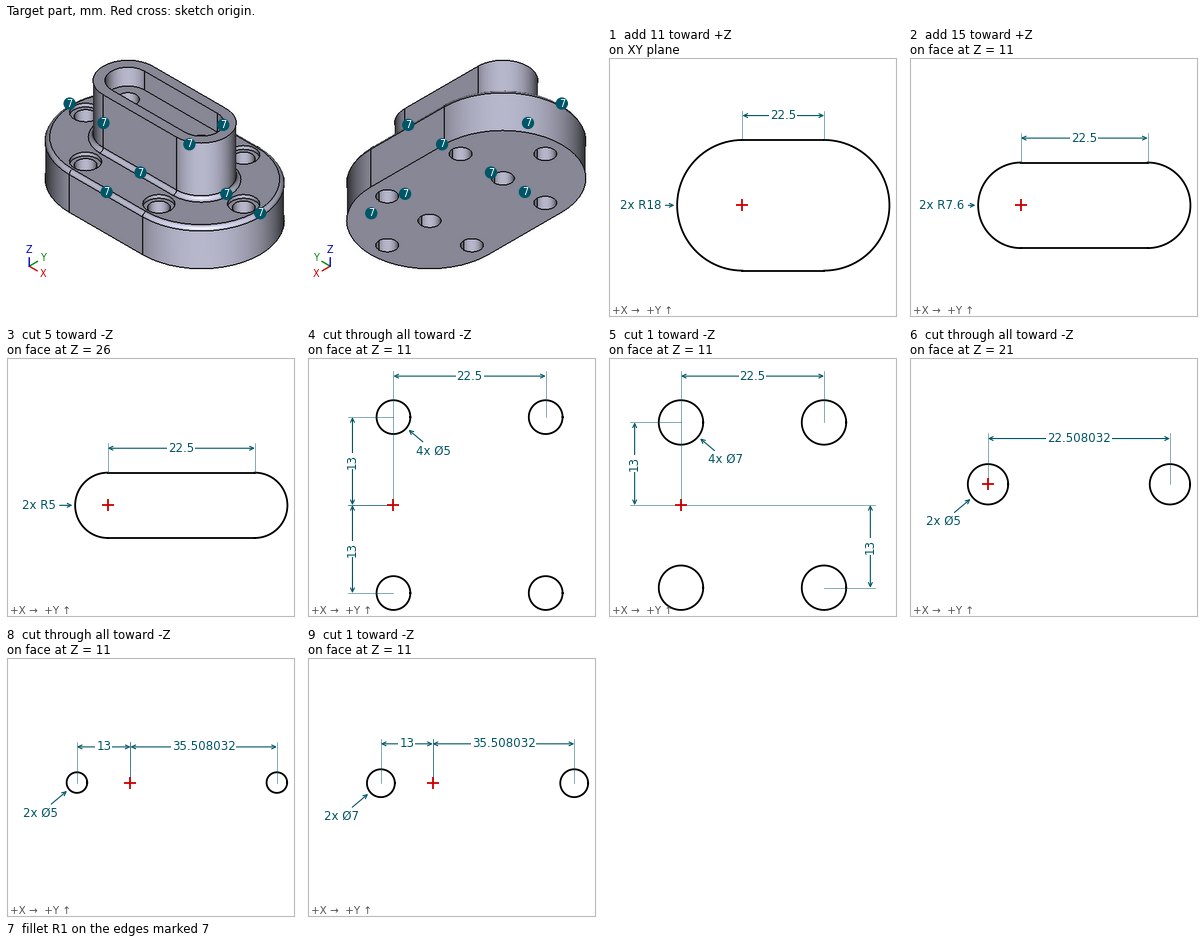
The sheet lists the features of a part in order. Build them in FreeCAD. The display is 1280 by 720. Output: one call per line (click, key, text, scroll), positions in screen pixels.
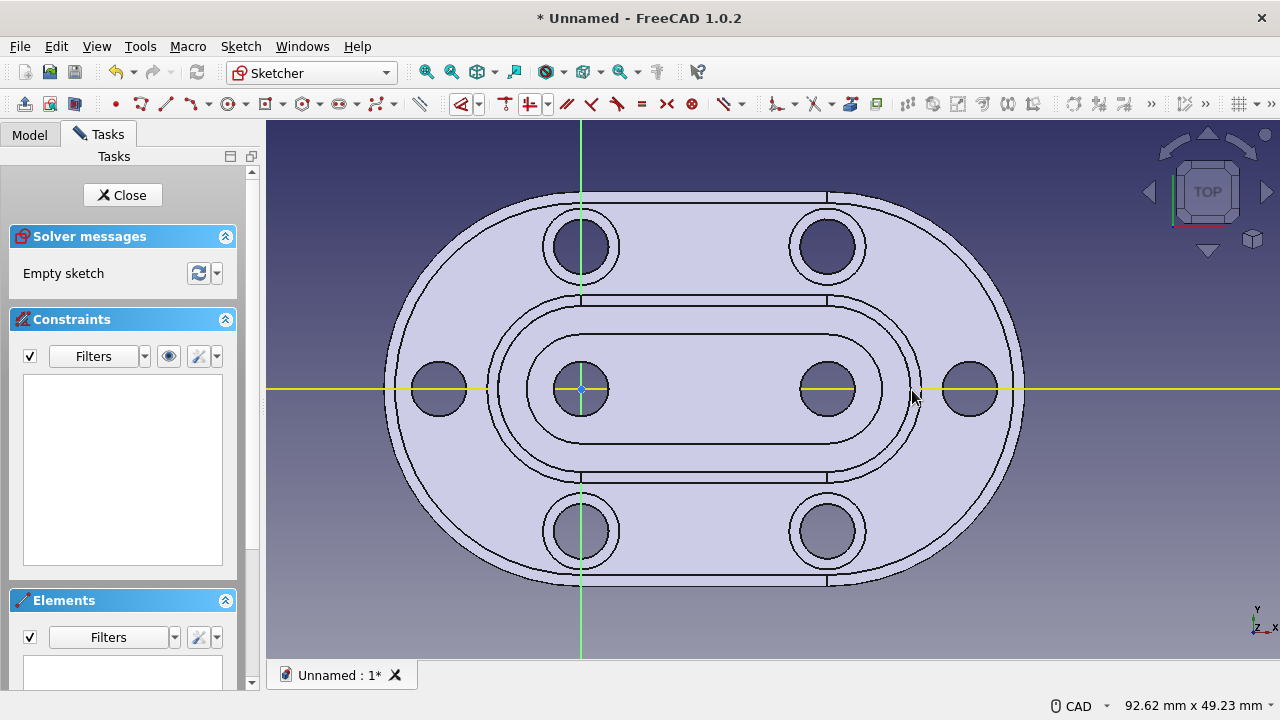
key(g)
key(c)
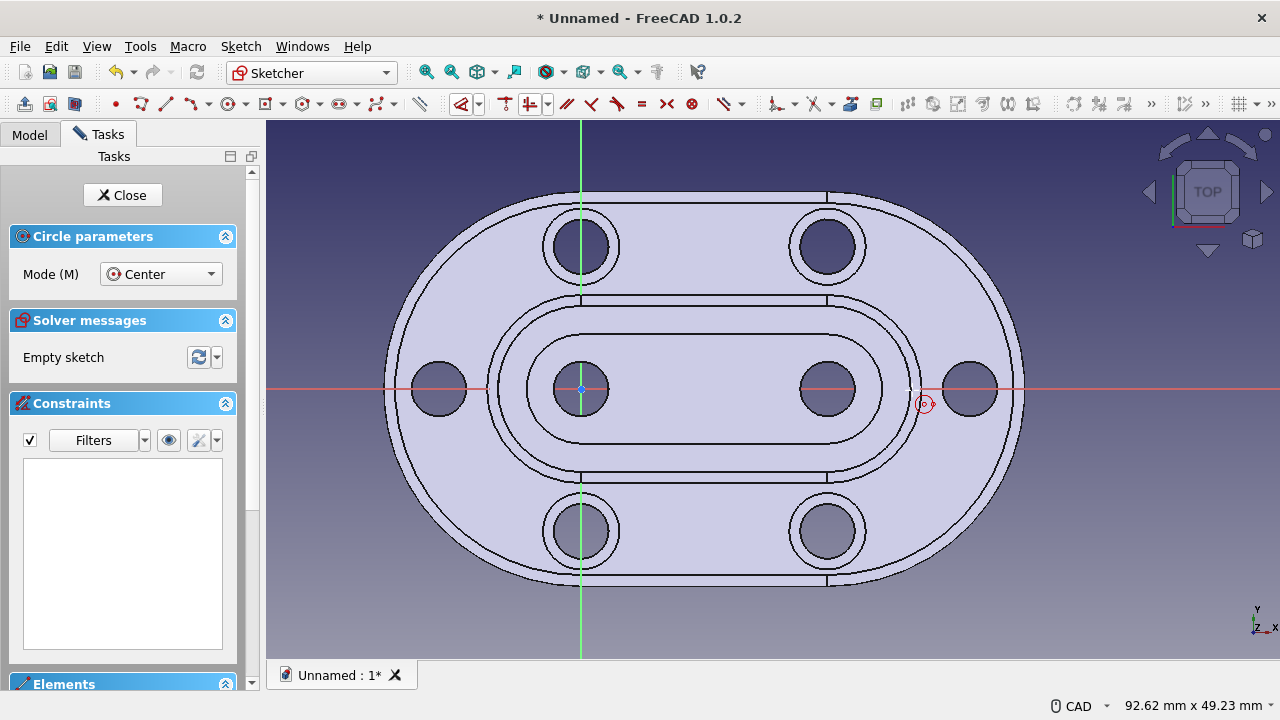
click(439, 389)
move(466, 362)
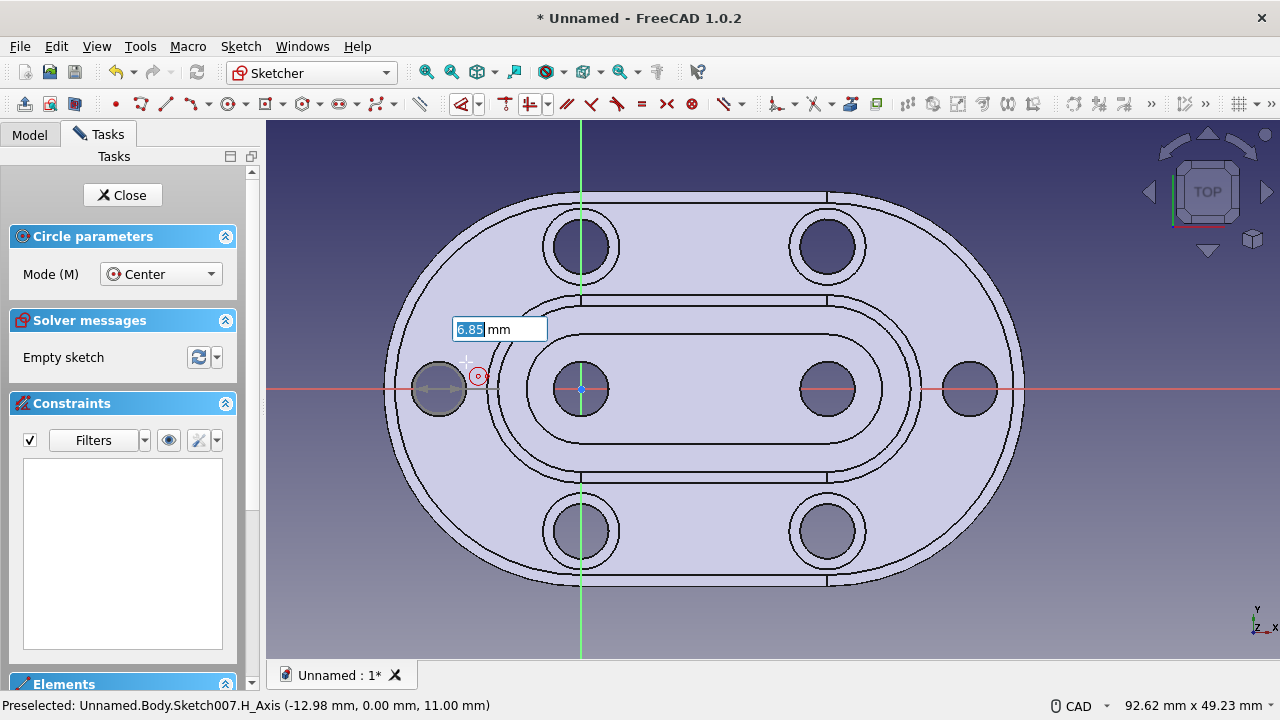
text(7)
key(Return)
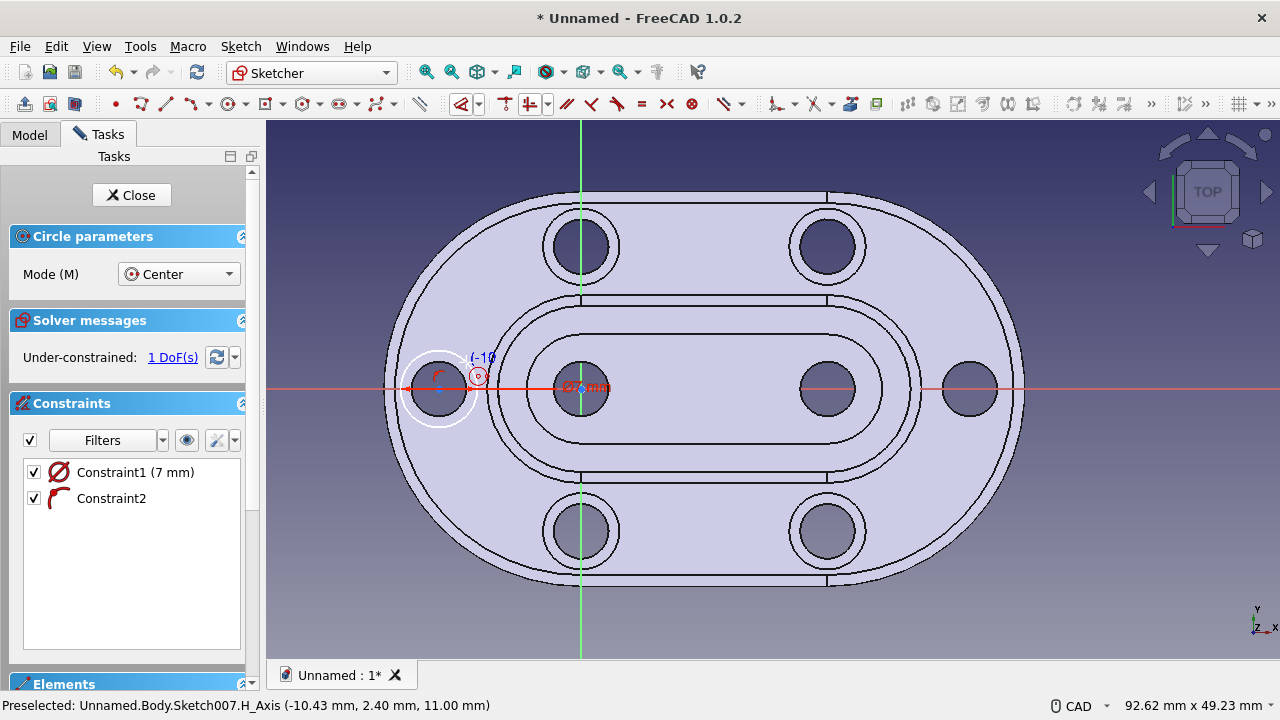
click(970, 389)
move(997, 362)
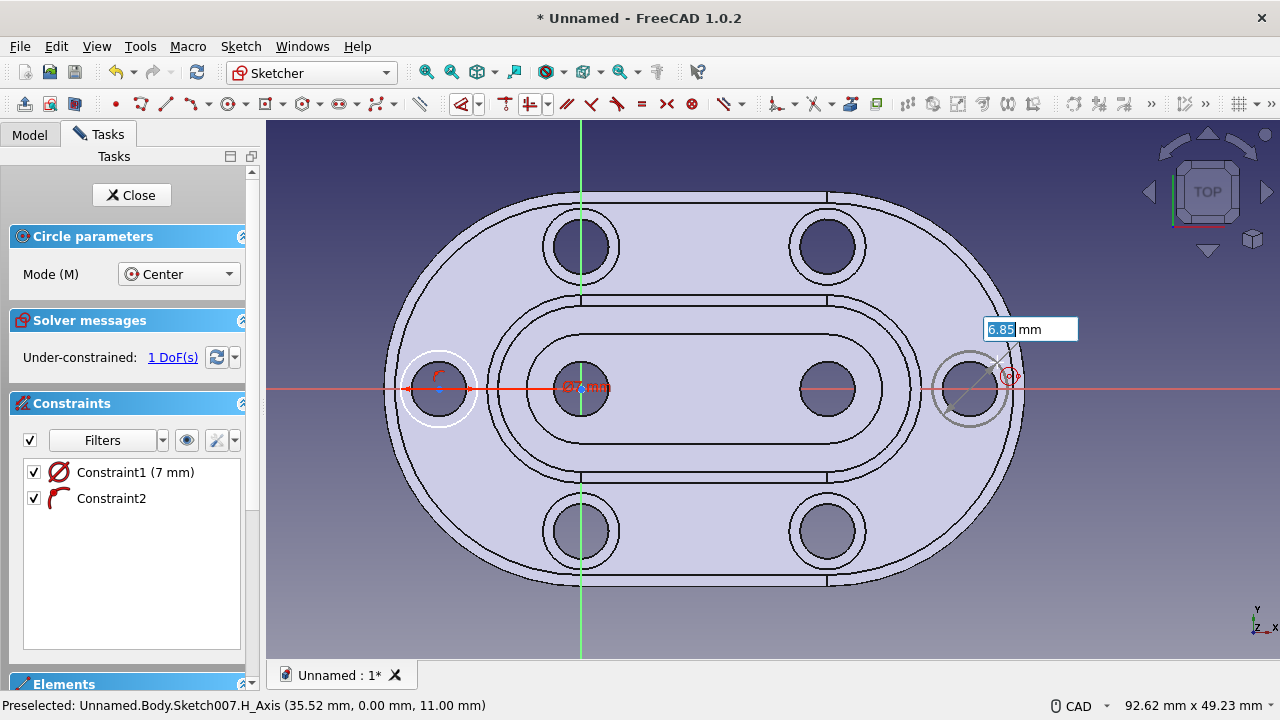
text(7)
key(Return)
key(Escape)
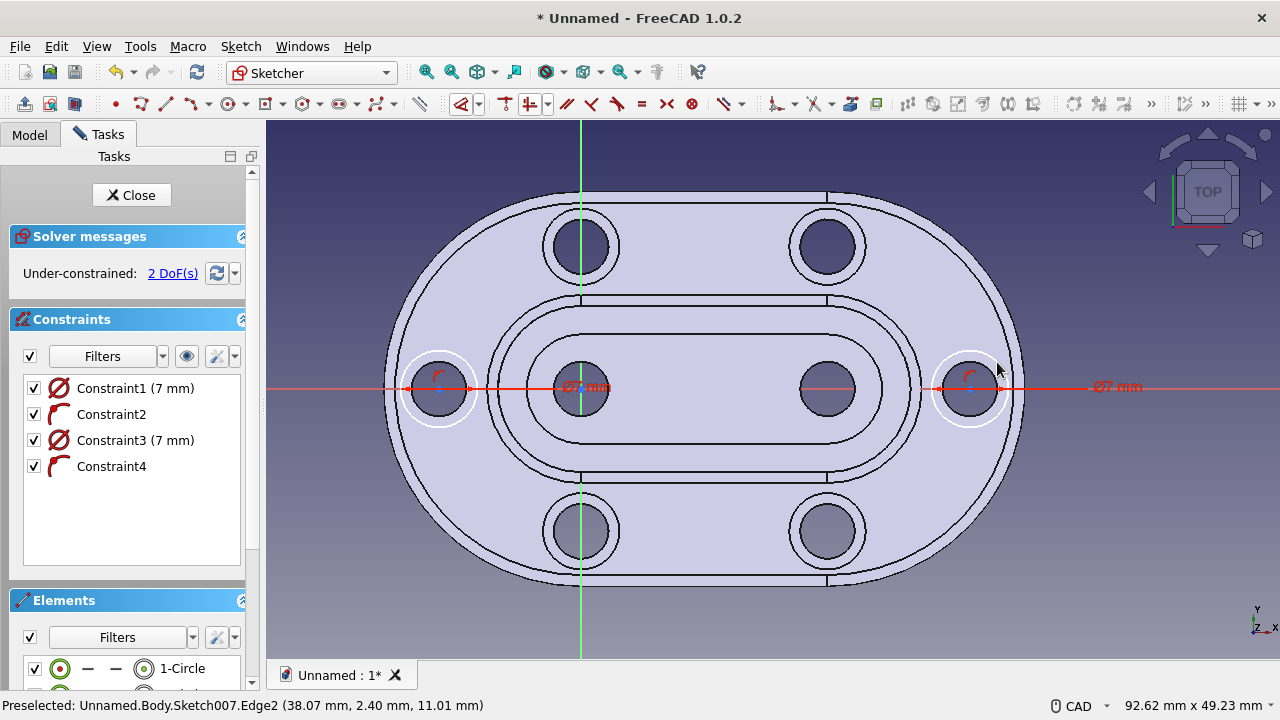
click(439, 389)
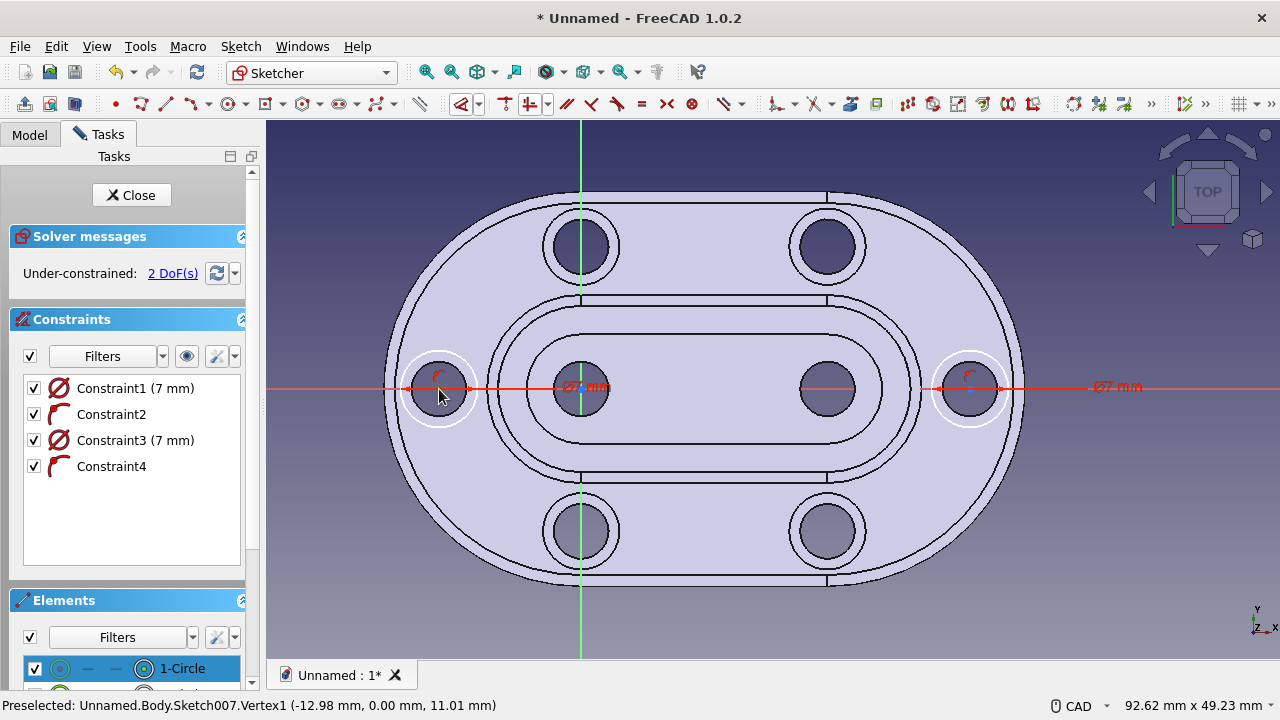
key(l)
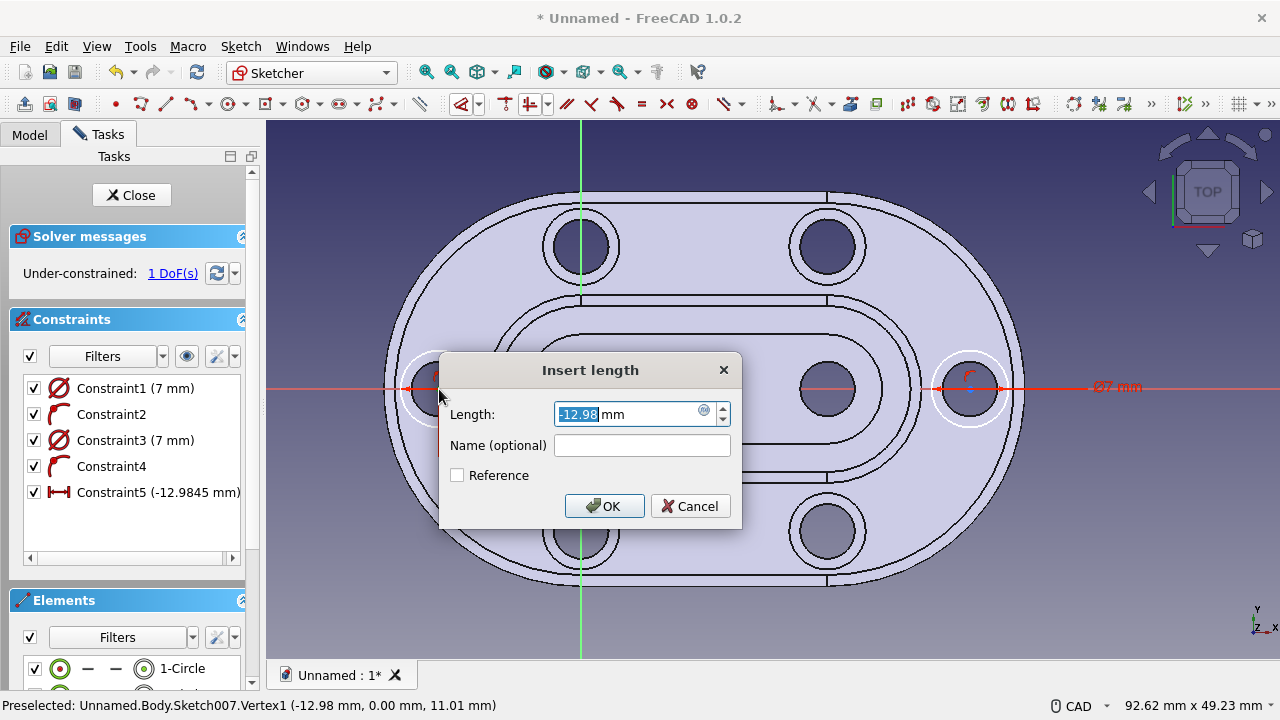
text(-13)
key(Return)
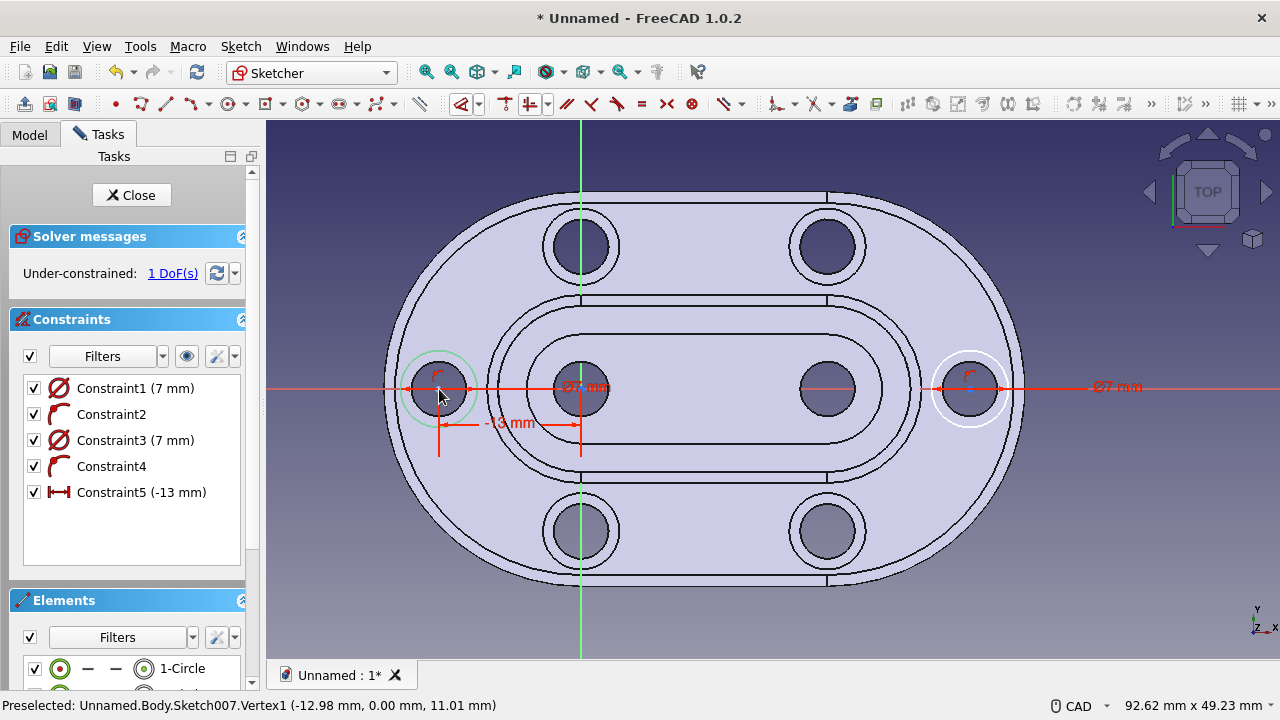
click(970, 389)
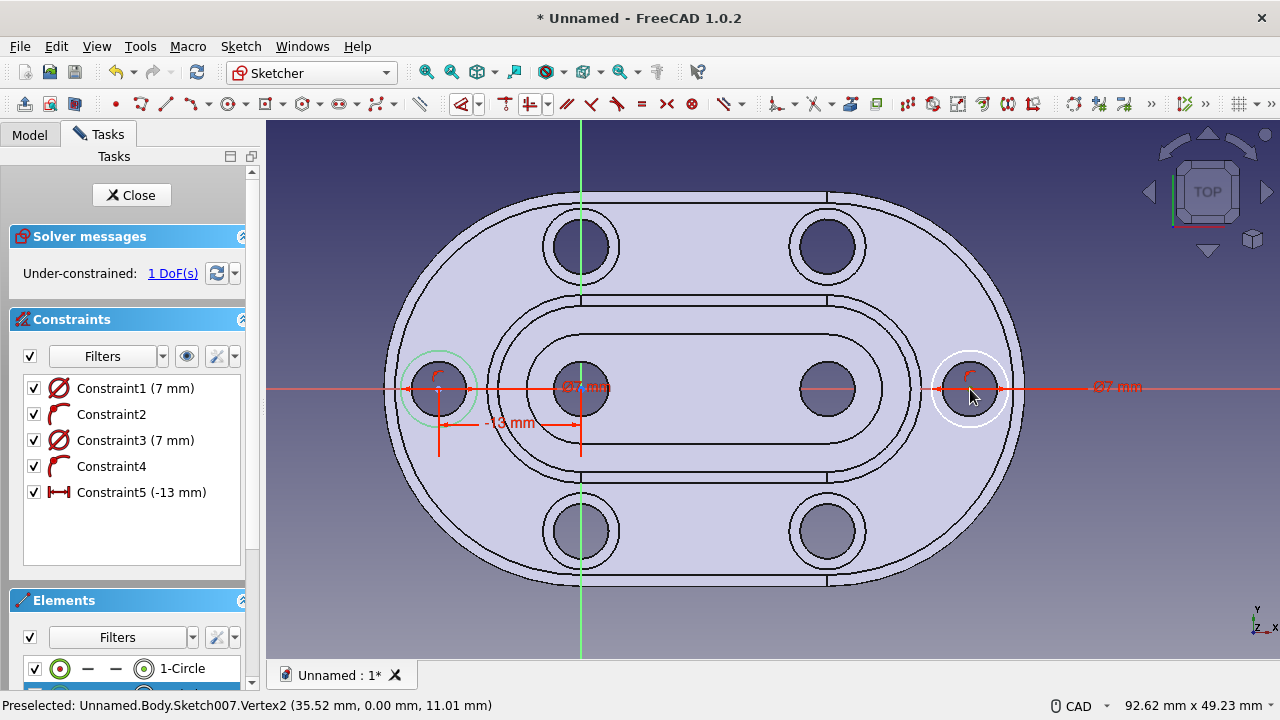
key(l)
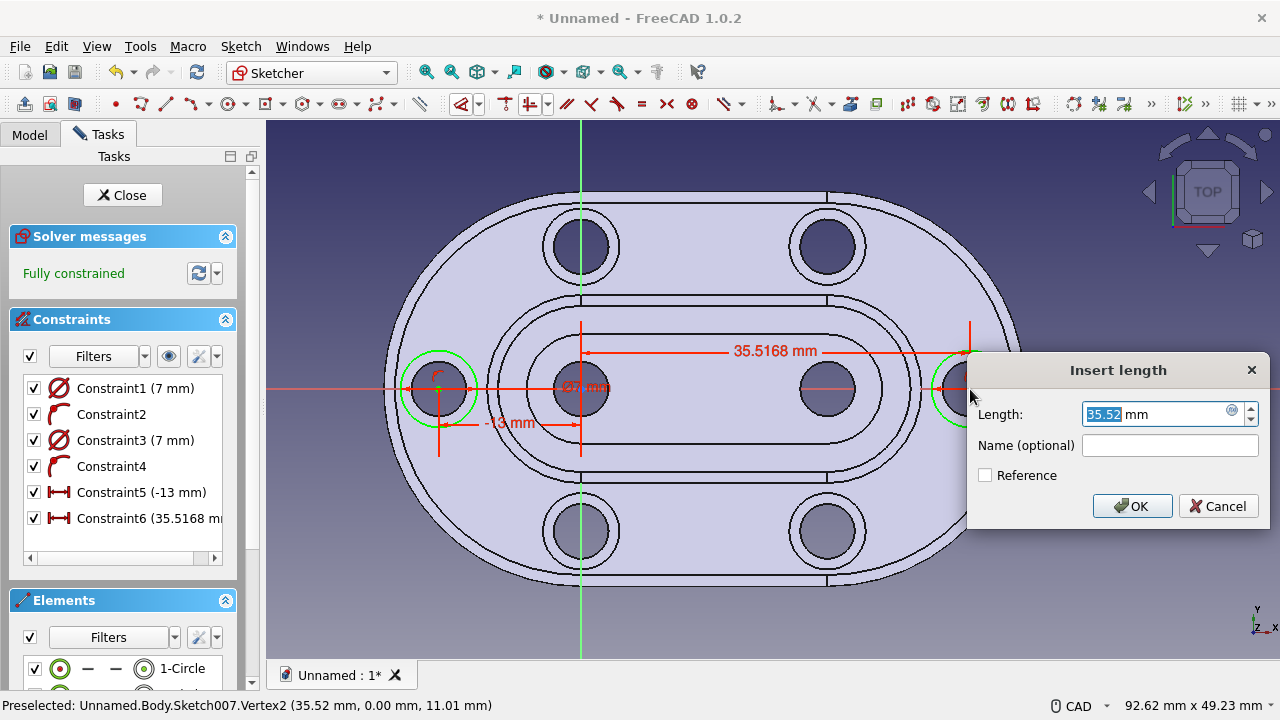
text(35.508032)
key(Return)